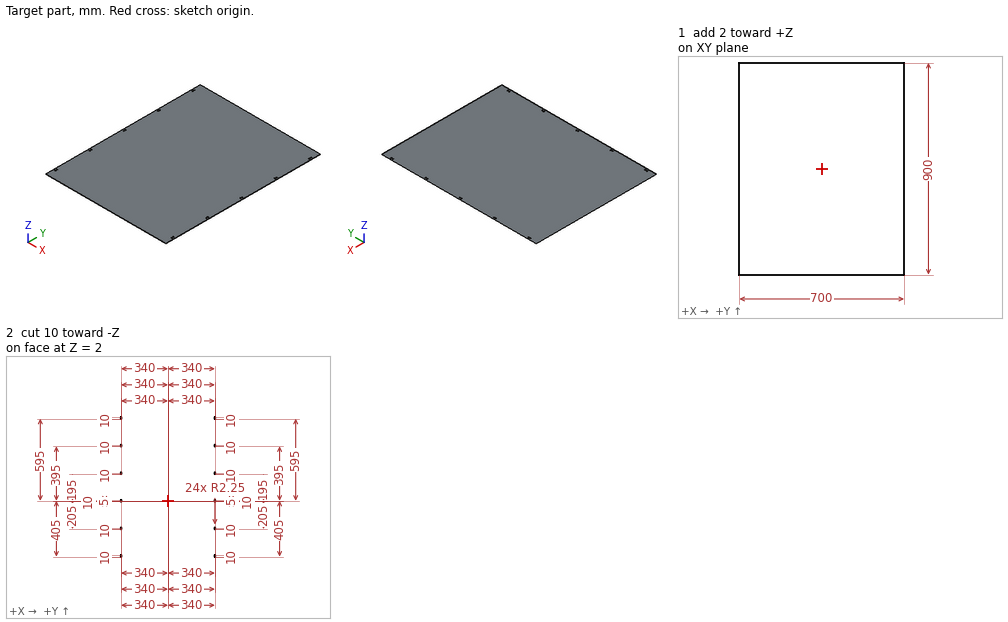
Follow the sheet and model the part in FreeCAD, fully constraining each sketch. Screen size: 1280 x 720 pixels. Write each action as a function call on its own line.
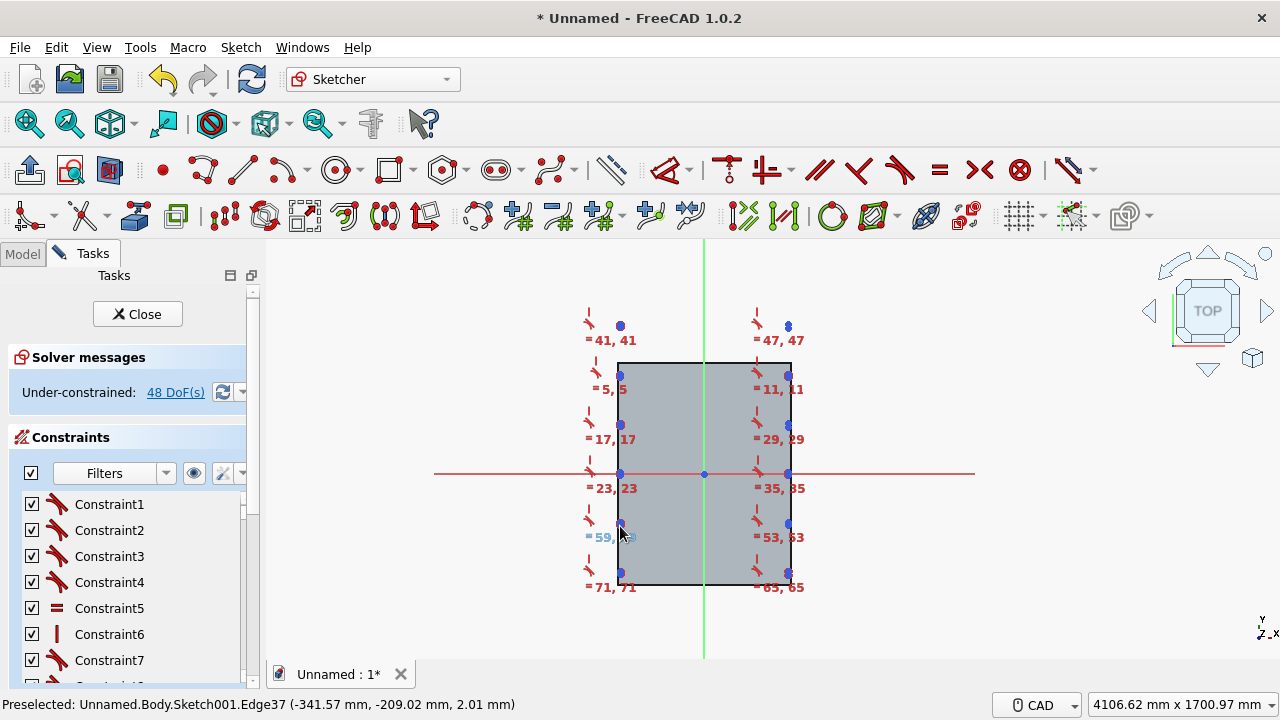
scroll(788, 576, up, 14)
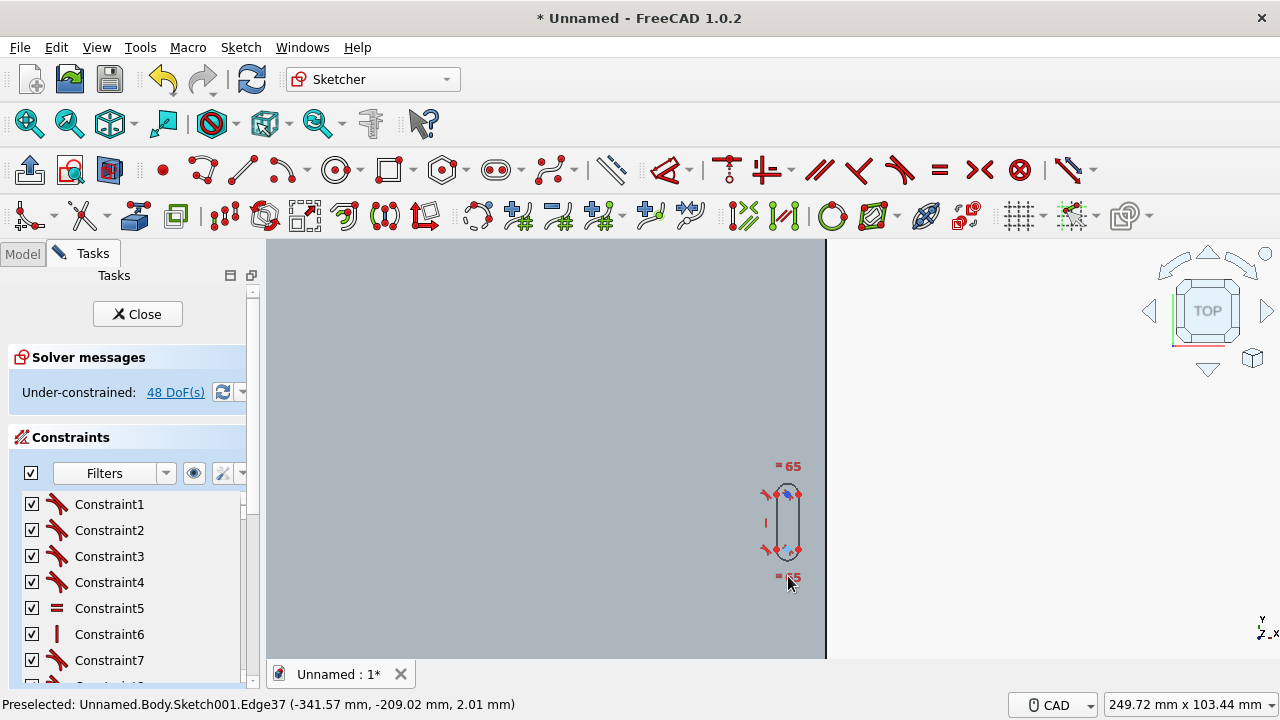
click(781, 559)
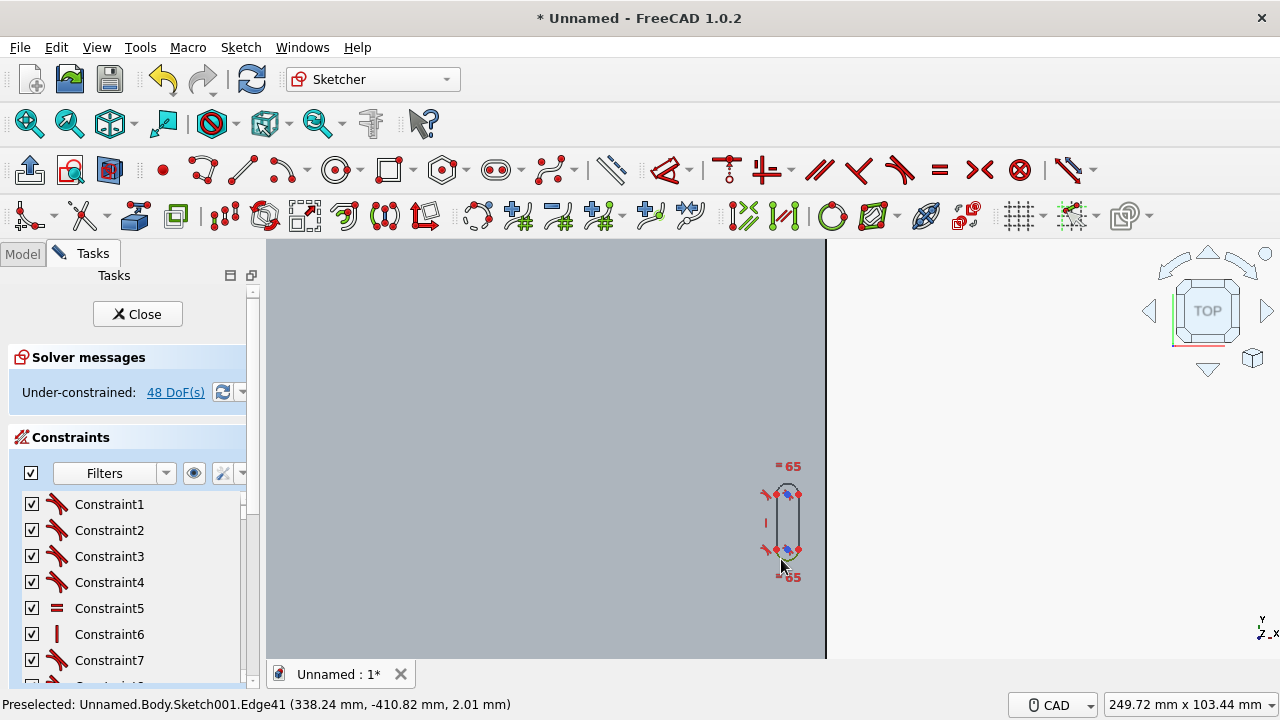
scroll(789, 576, down, 14)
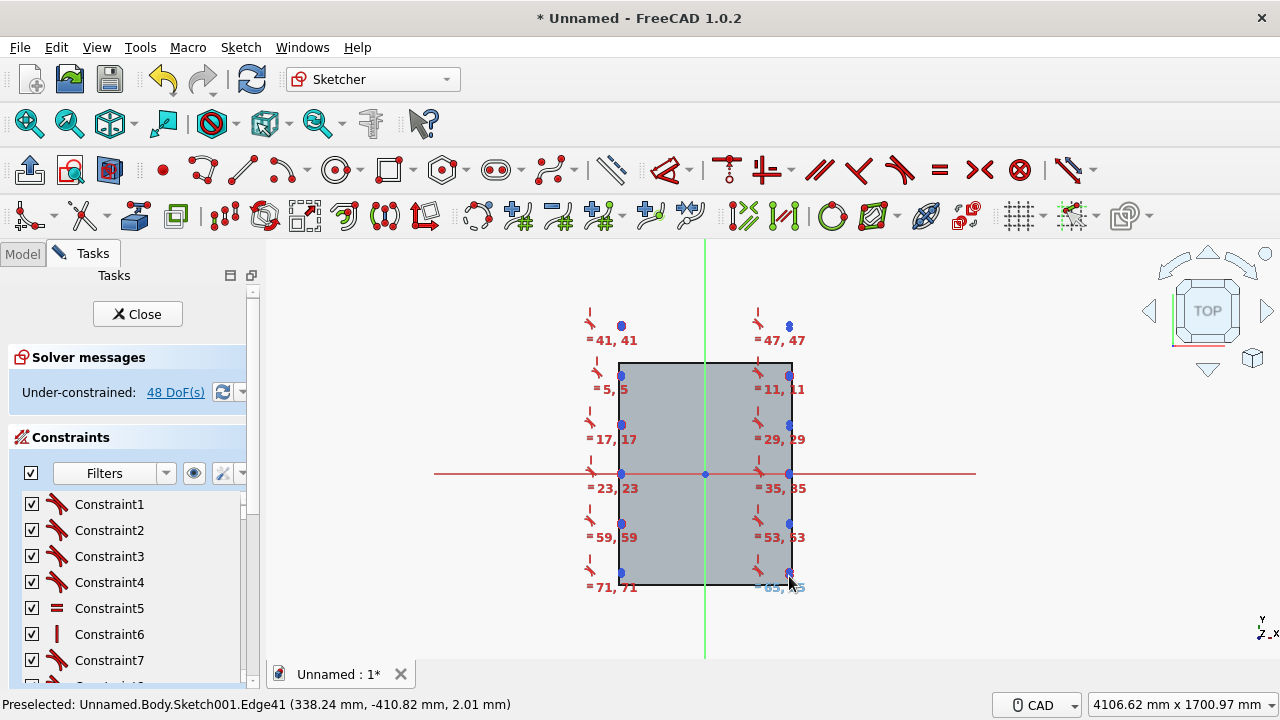
scroll(622, 575, up, 14)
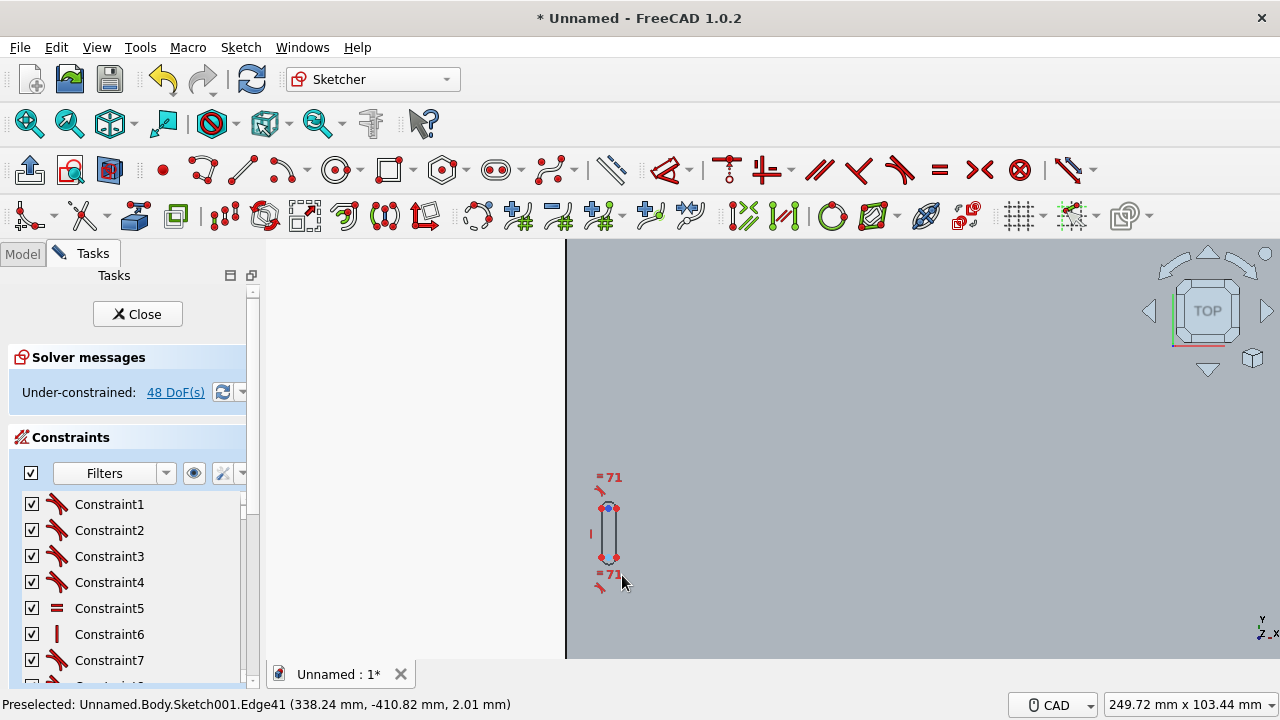
click(609, 565)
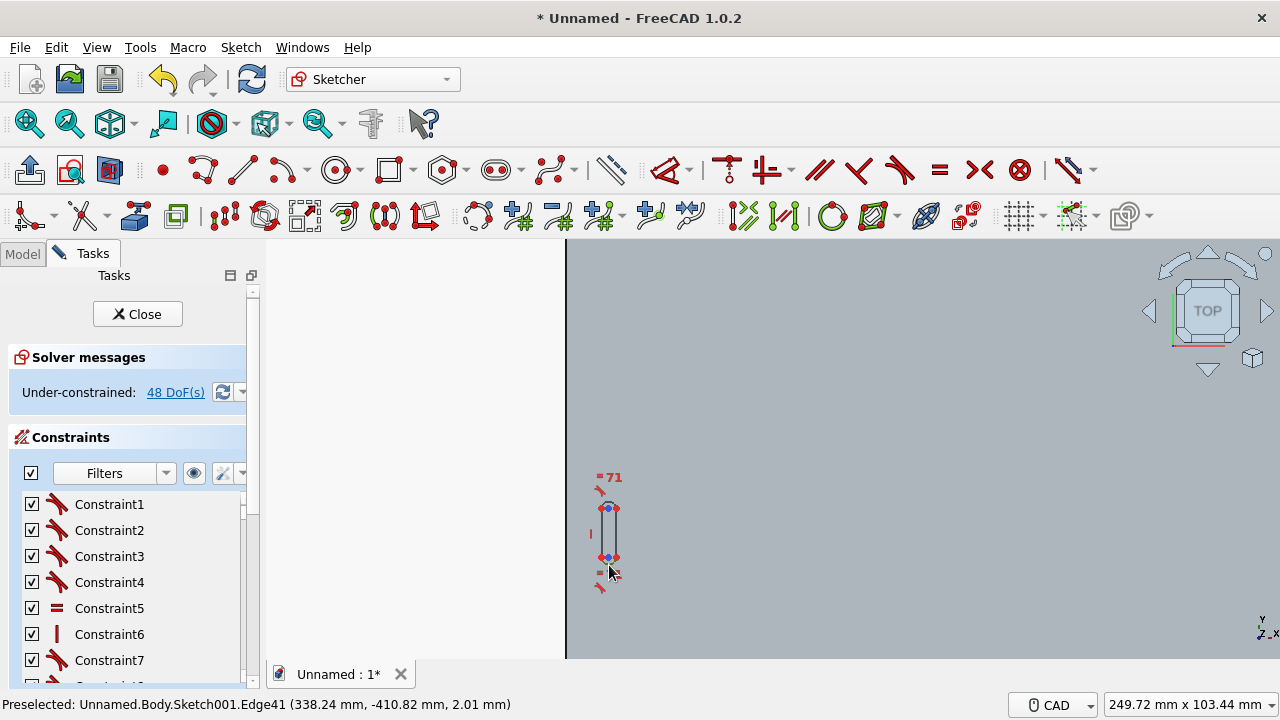
click(940, 170)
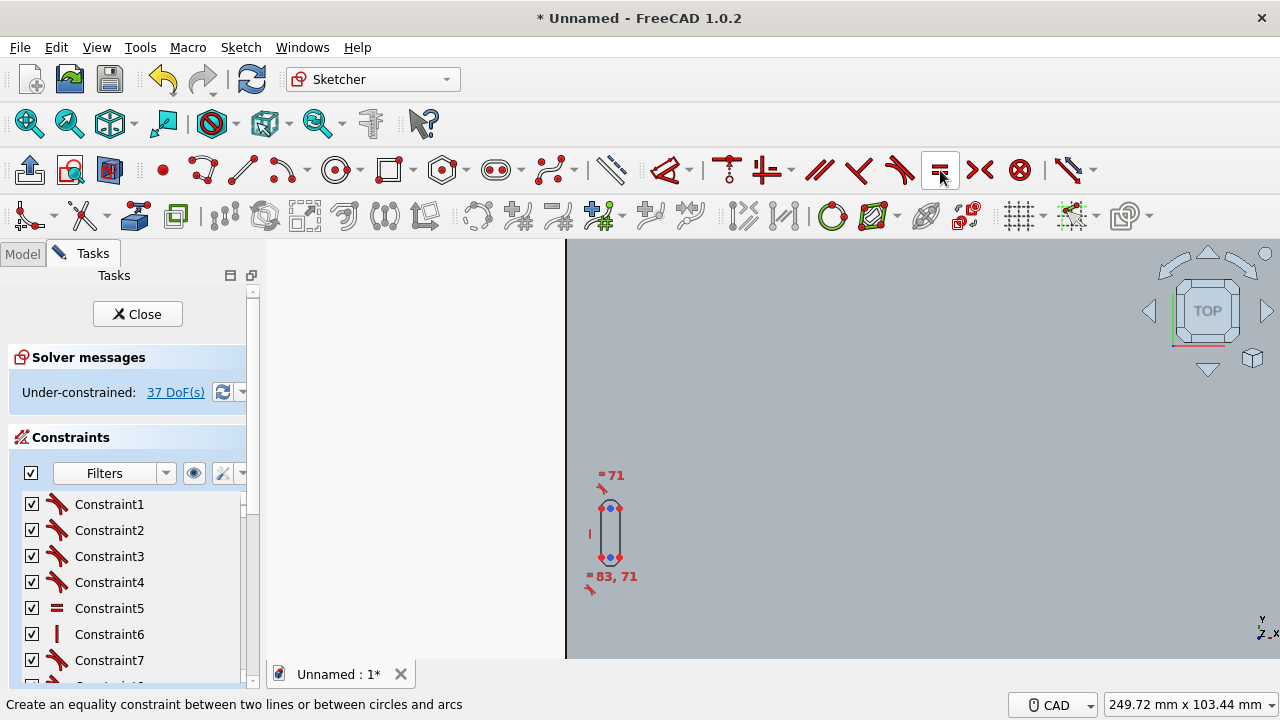
click(666, 170)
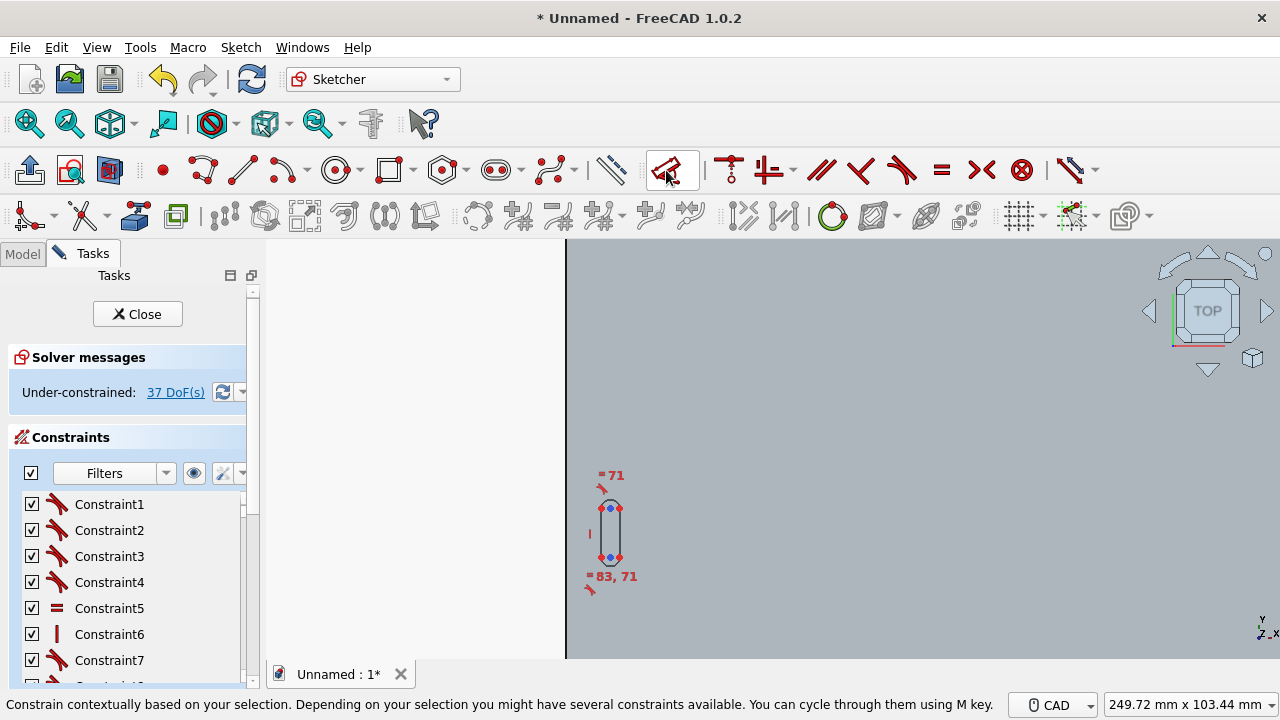
scroll(621, 575, down, 14)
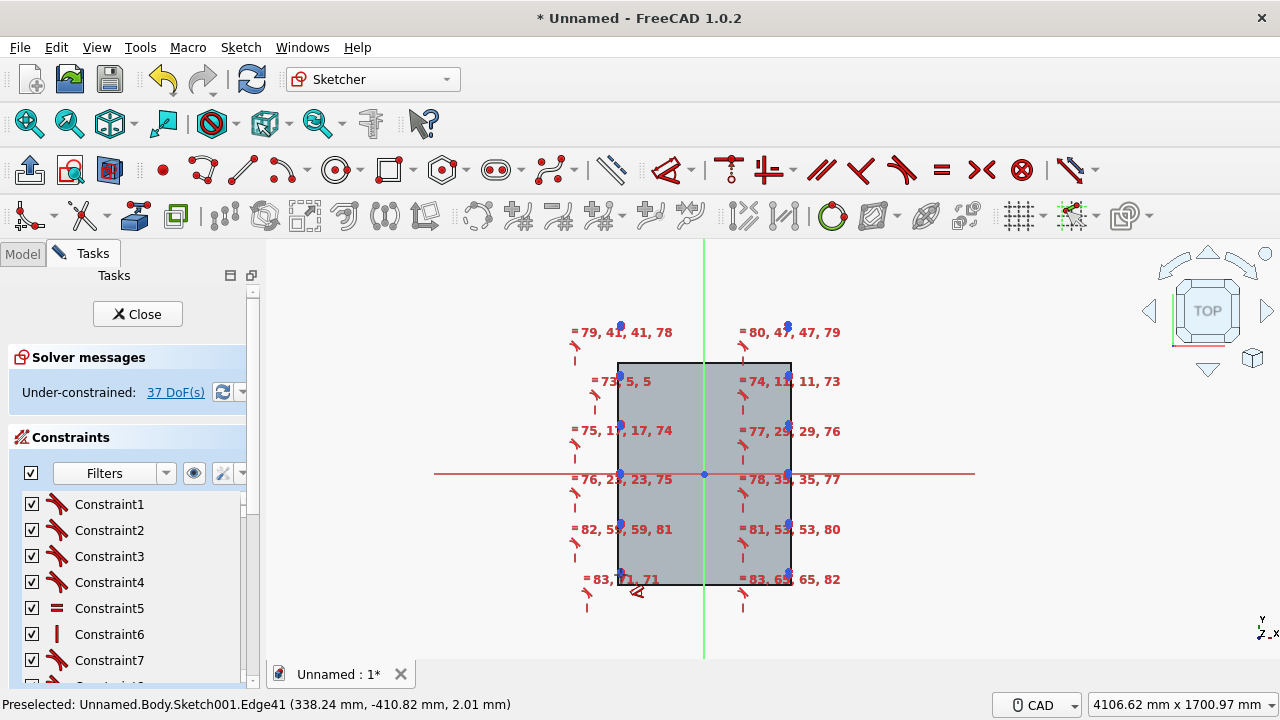
scroll(620, 377, up, 14)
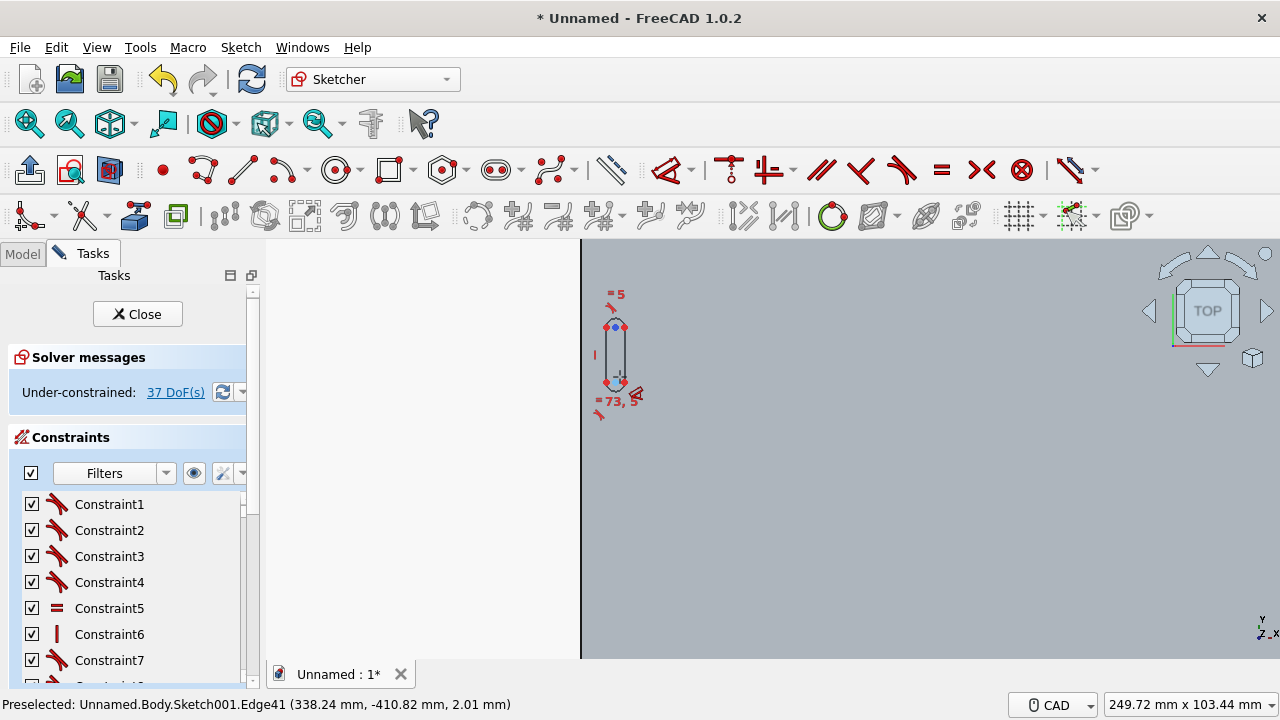
click(606, 366)
click(572, 355)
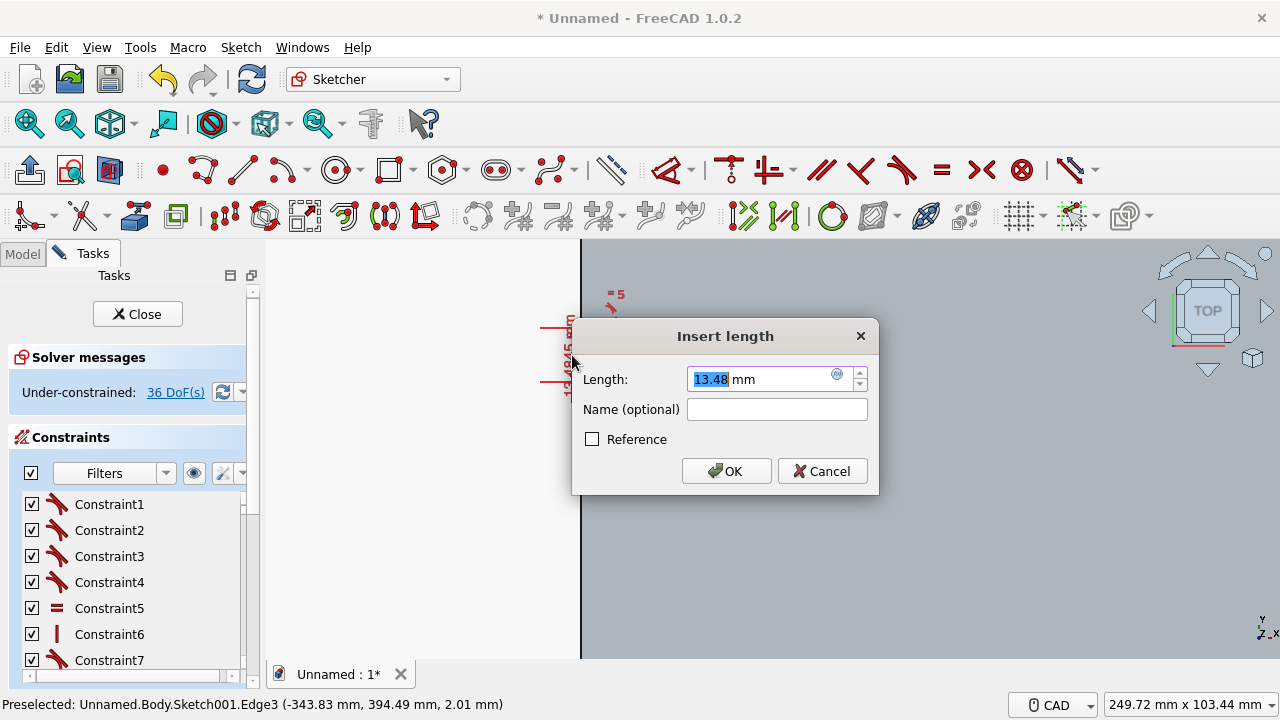
text(10)
key(Return)